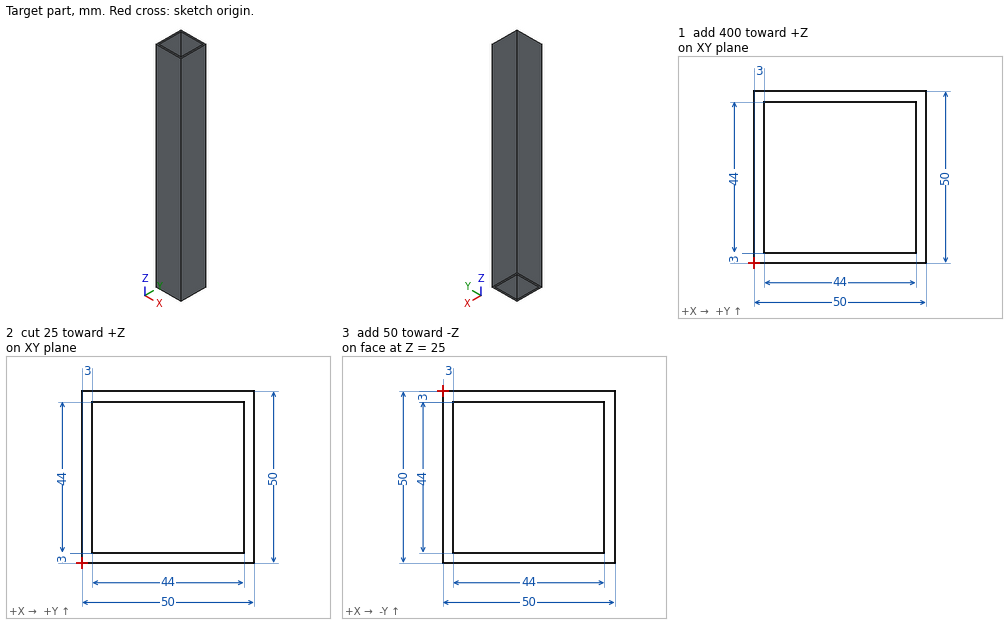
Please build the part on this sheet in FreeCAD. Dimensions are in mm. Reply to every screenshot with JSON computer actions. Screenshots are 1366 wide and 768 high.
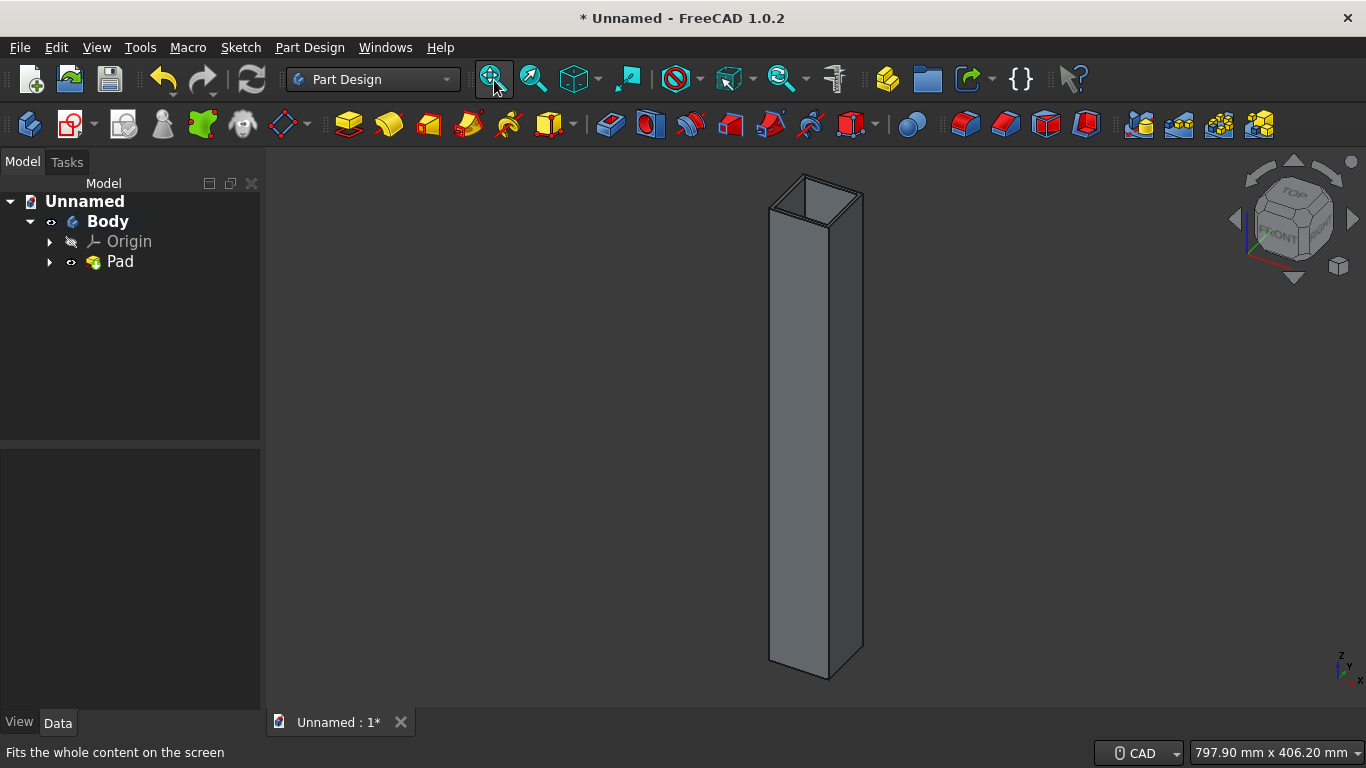
{"action": "left_click", "coordinate": [70, 124]}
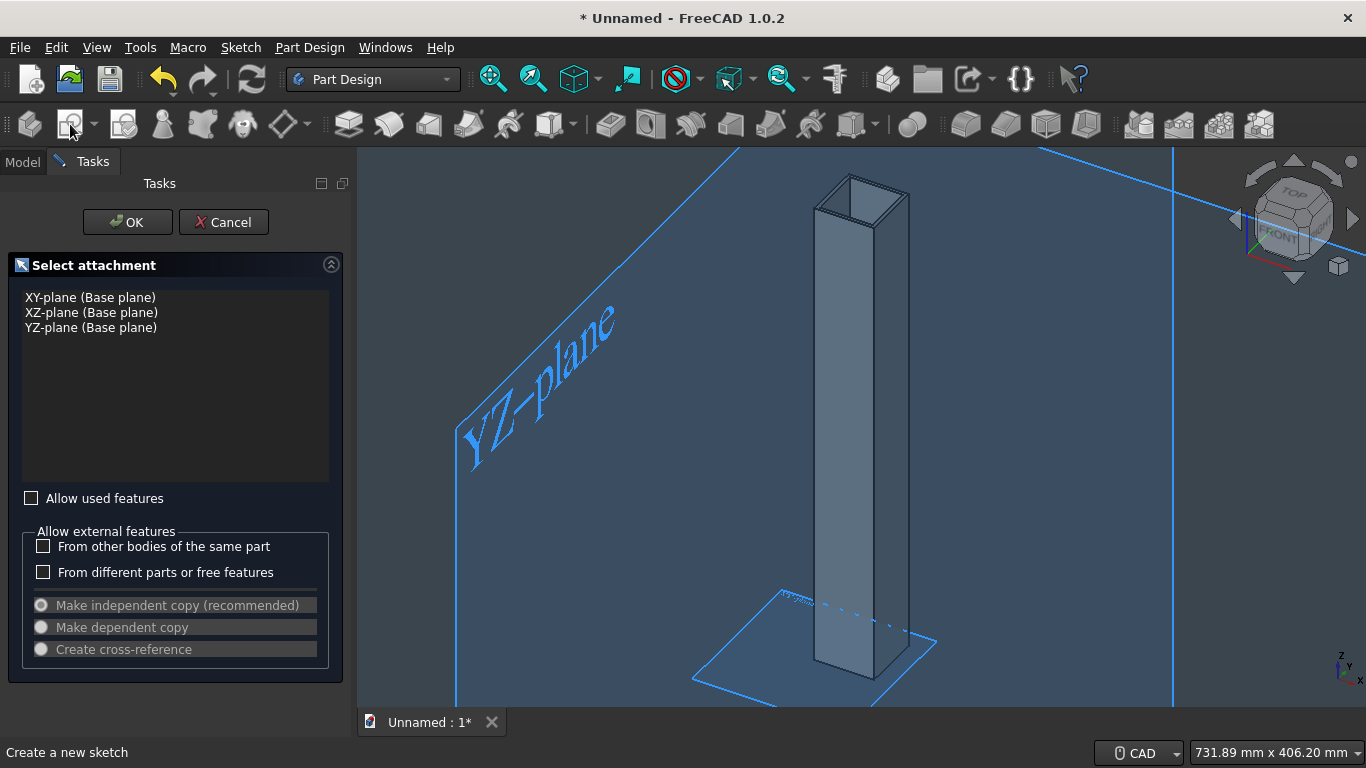
{"action": "left_click", "coordinate": [82, 298]}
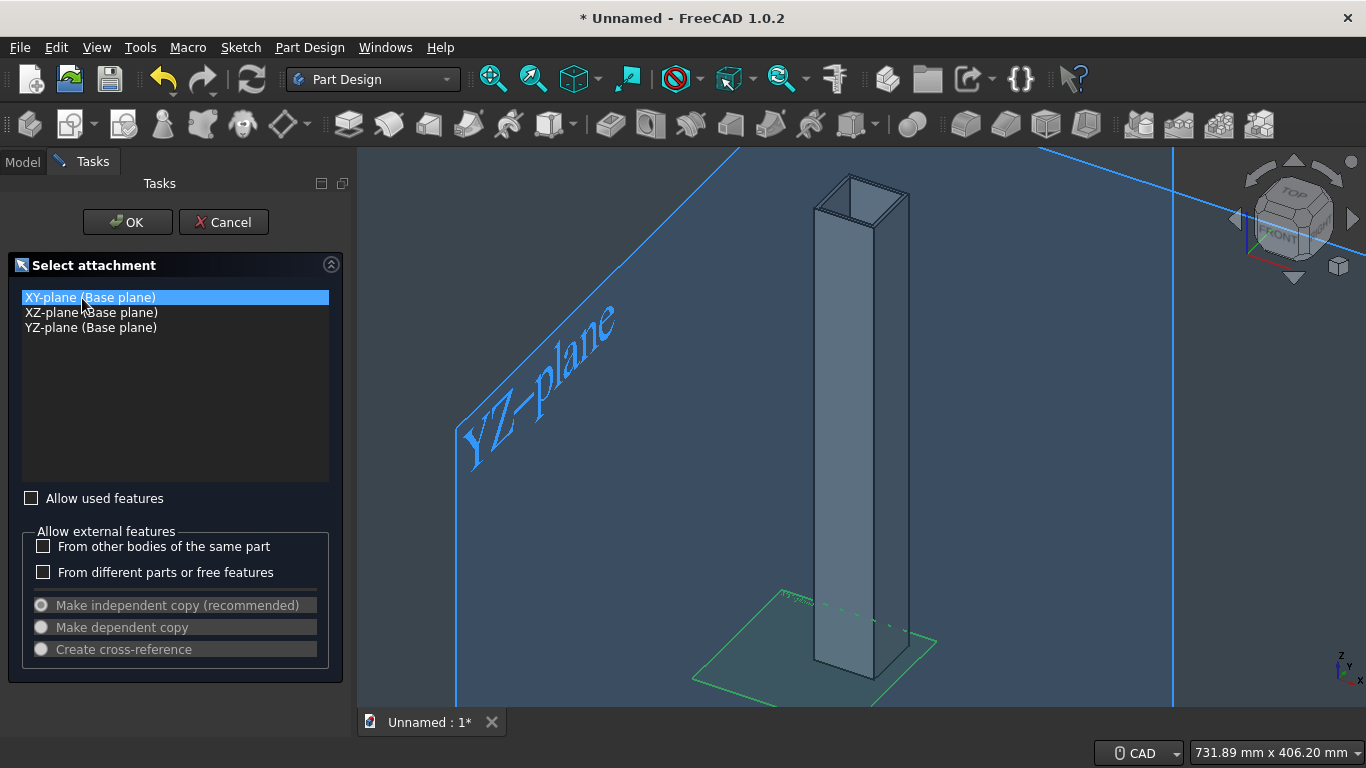
{"action": "left_click", "coordinate": [128, 222]}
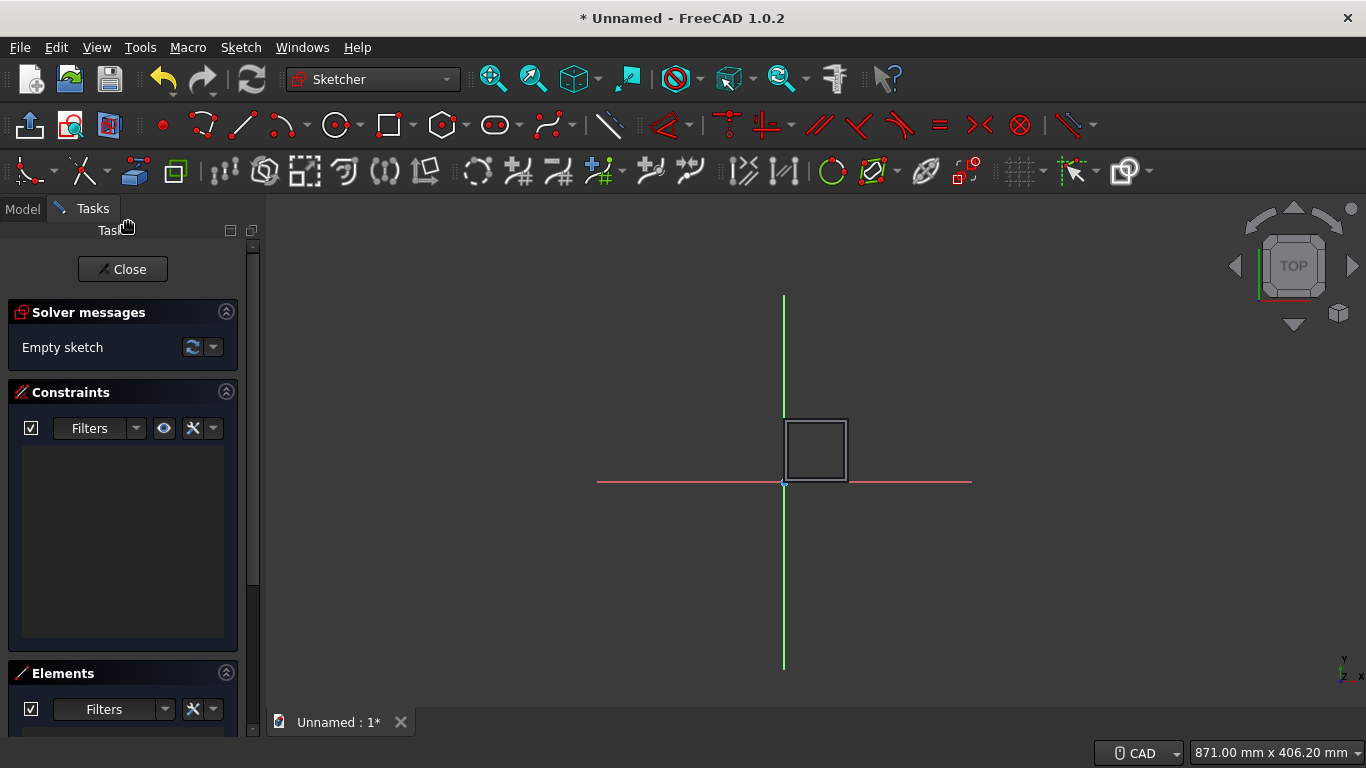
{"action": "left_click", "coordinate": [110, 126]}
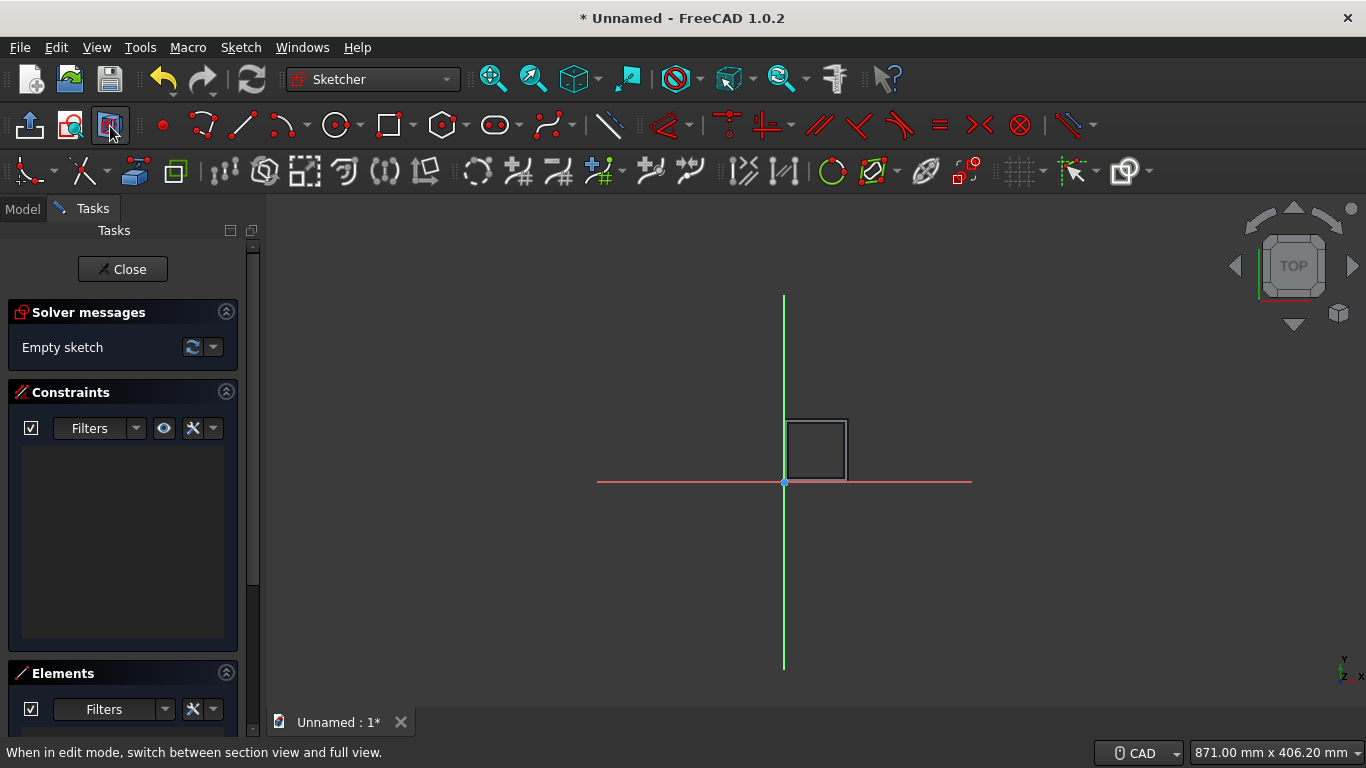
{"action": "scroll", "coordinate": [833, 450], "scroll_direction": "up", "scroll_amount": 8}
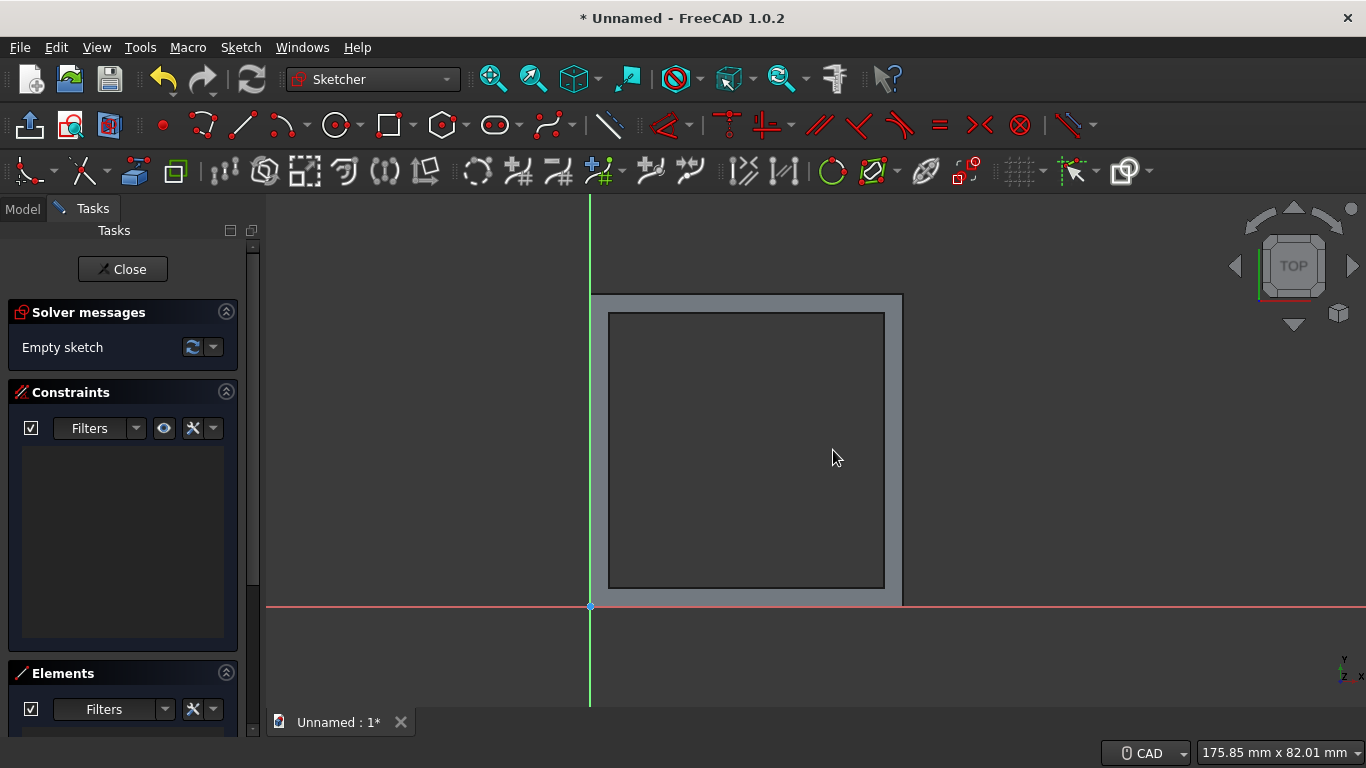
{"action": "left_click", "coordinate": [390, 126]}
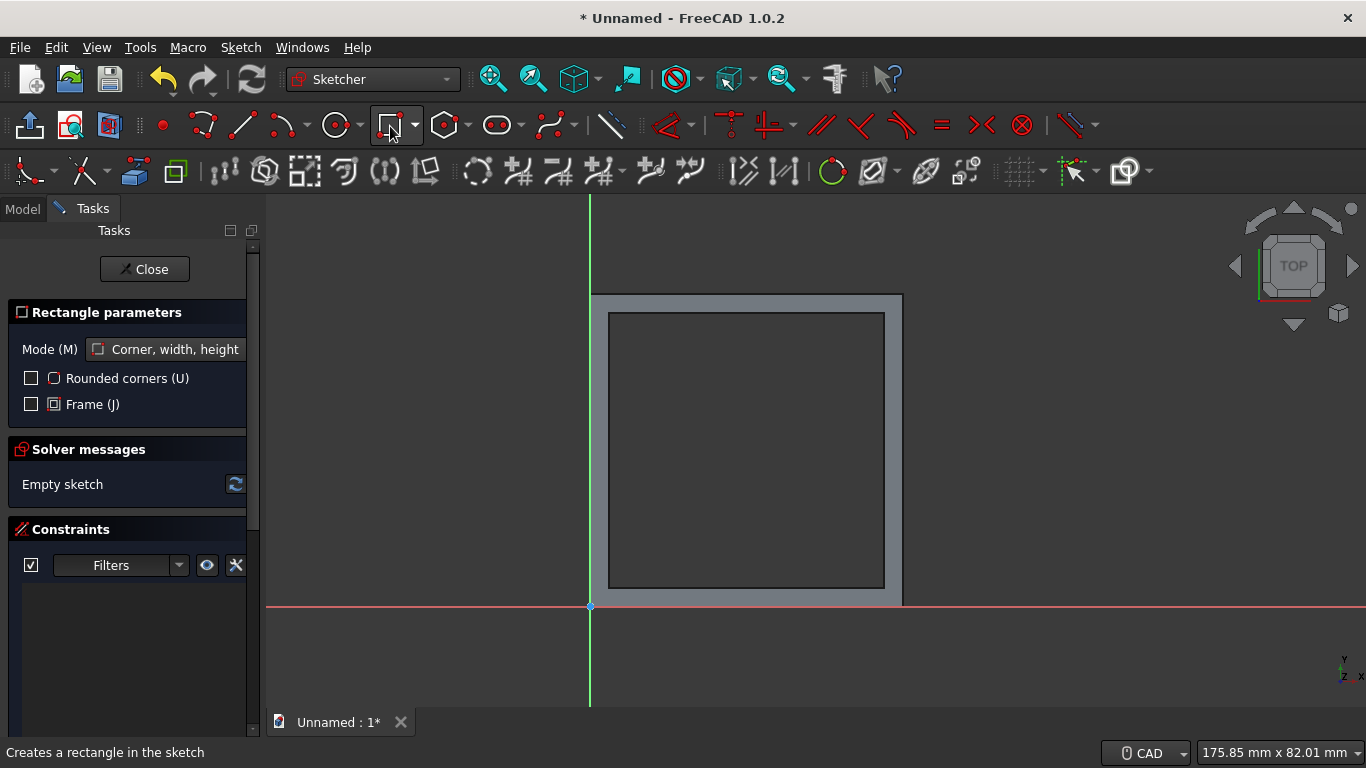
{"action": "left_click", "coordinate": [590, 607]}
{"action": "left_click", "coordinate": [903, 294]}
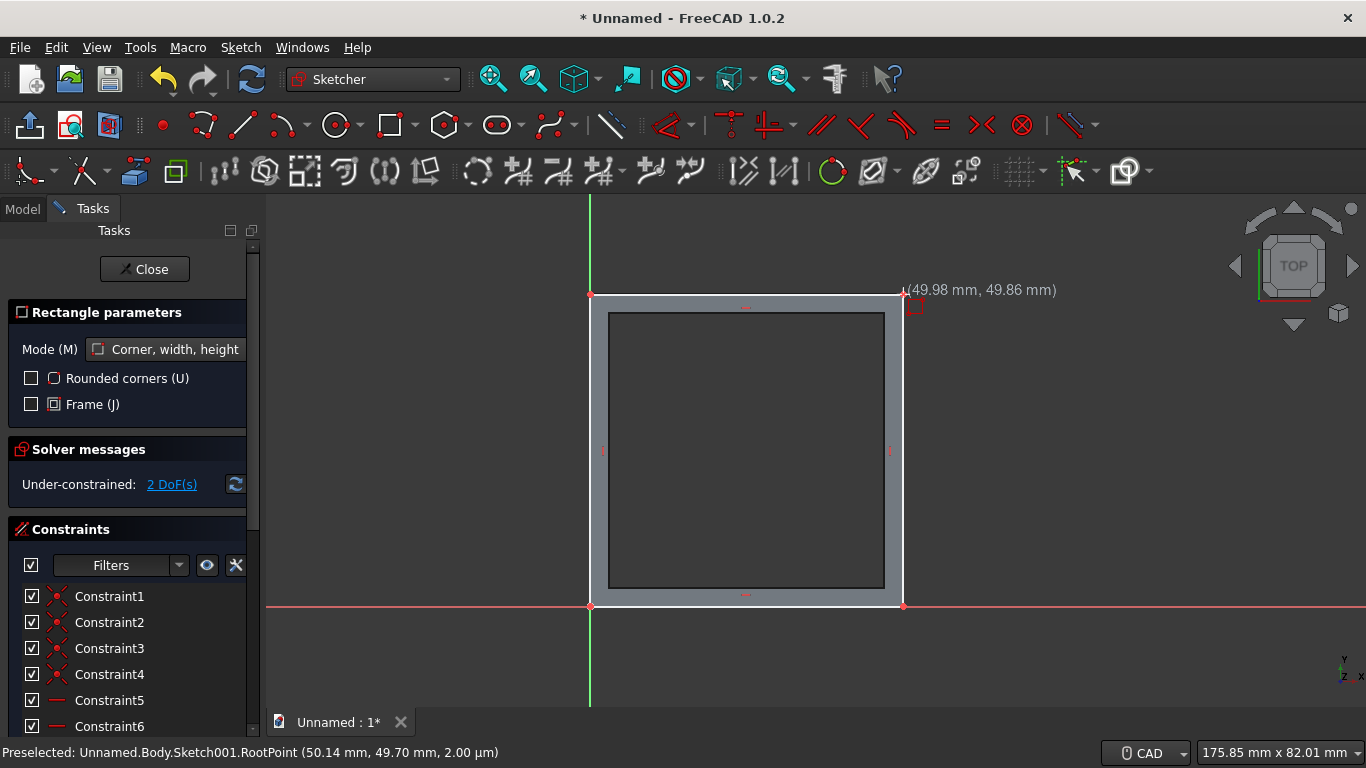
{"action": "left_click", "coordinate": [609, 313]}
{"action": "left_click", "coordinate": [884, 588]}
{"action": "key", "text": "Escape"}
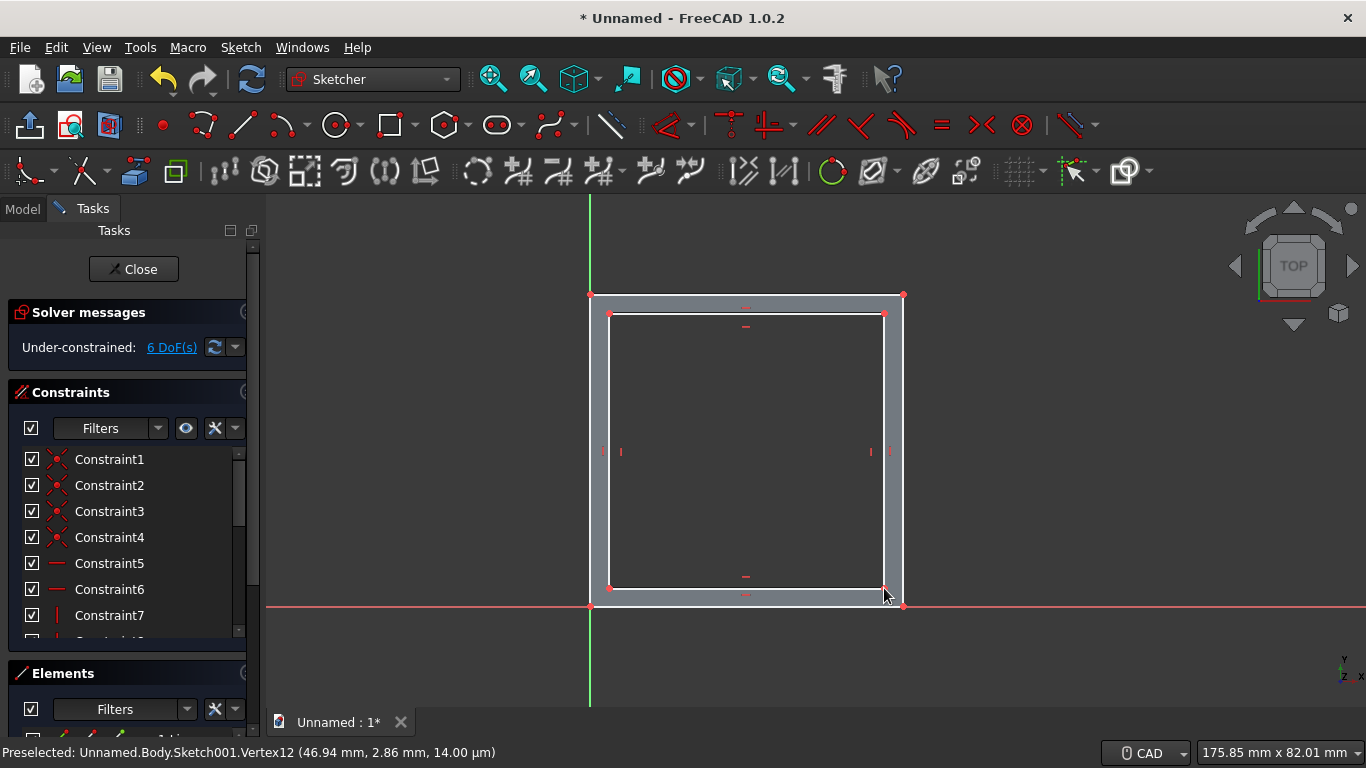
{"action": "left_click", "coordinate": [666, 126]}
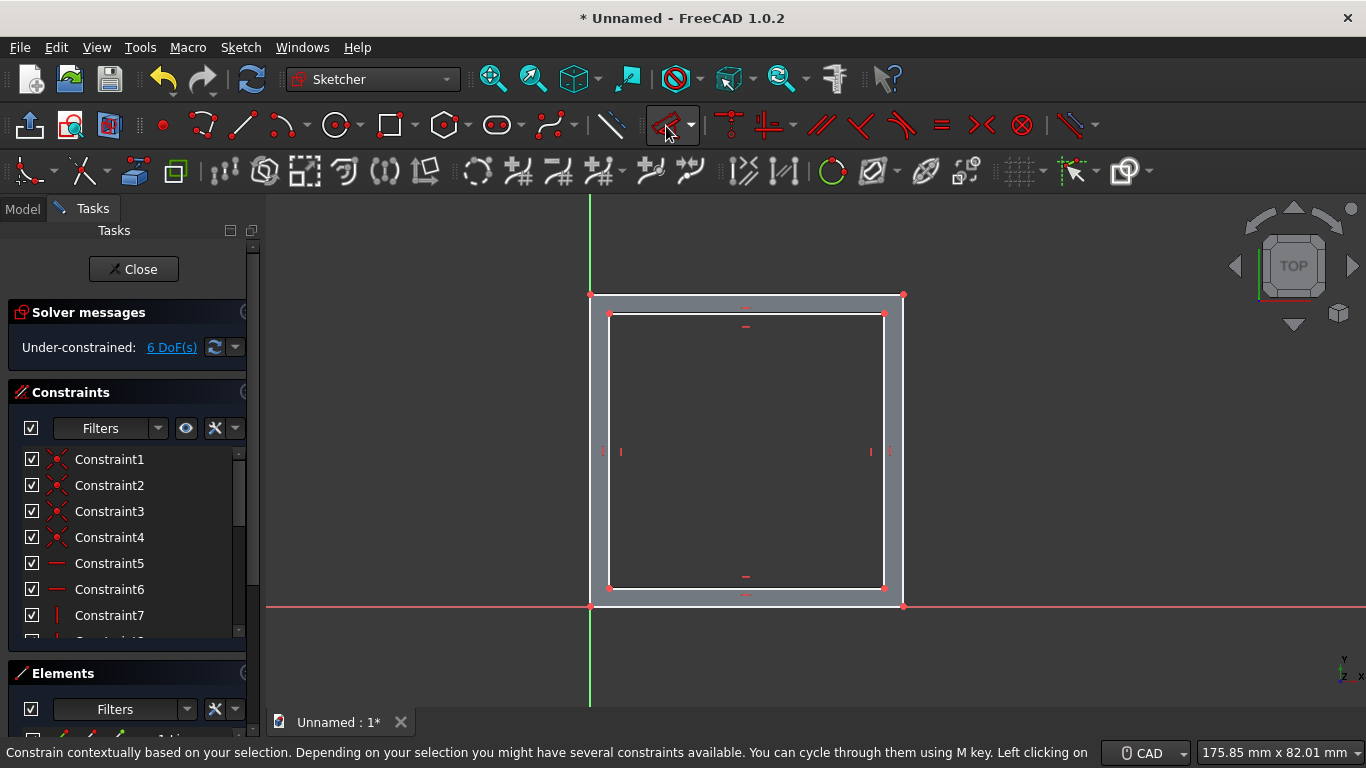
{"action": "left_click", "coordinate": [684, 607]}
{"action": "left_click", "coordinate": [747, 641]}